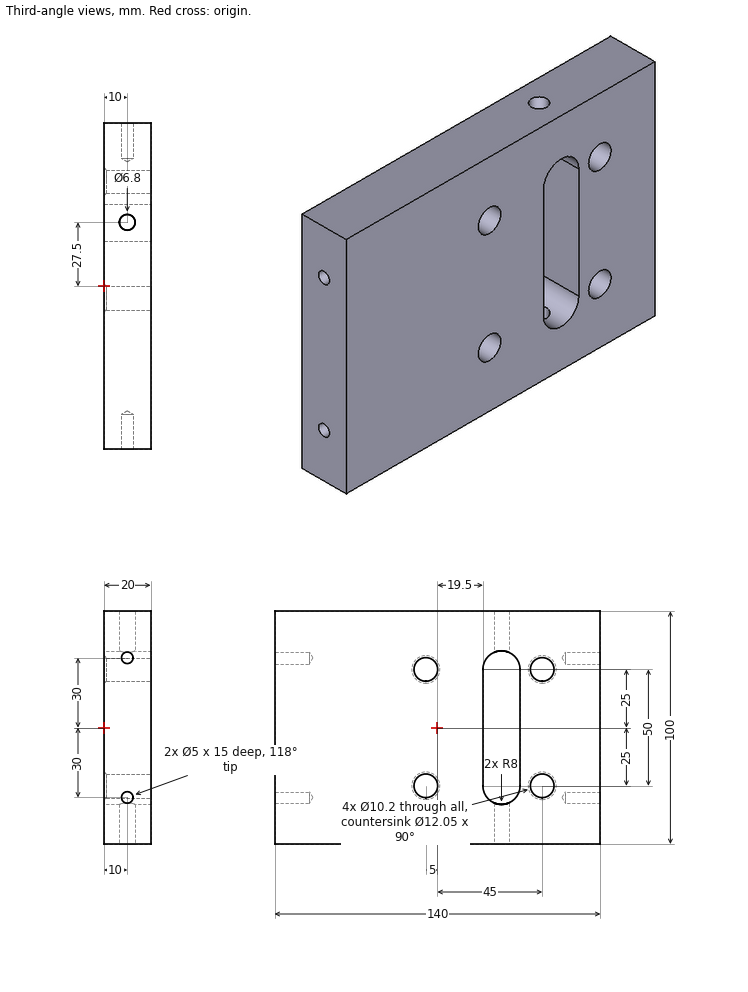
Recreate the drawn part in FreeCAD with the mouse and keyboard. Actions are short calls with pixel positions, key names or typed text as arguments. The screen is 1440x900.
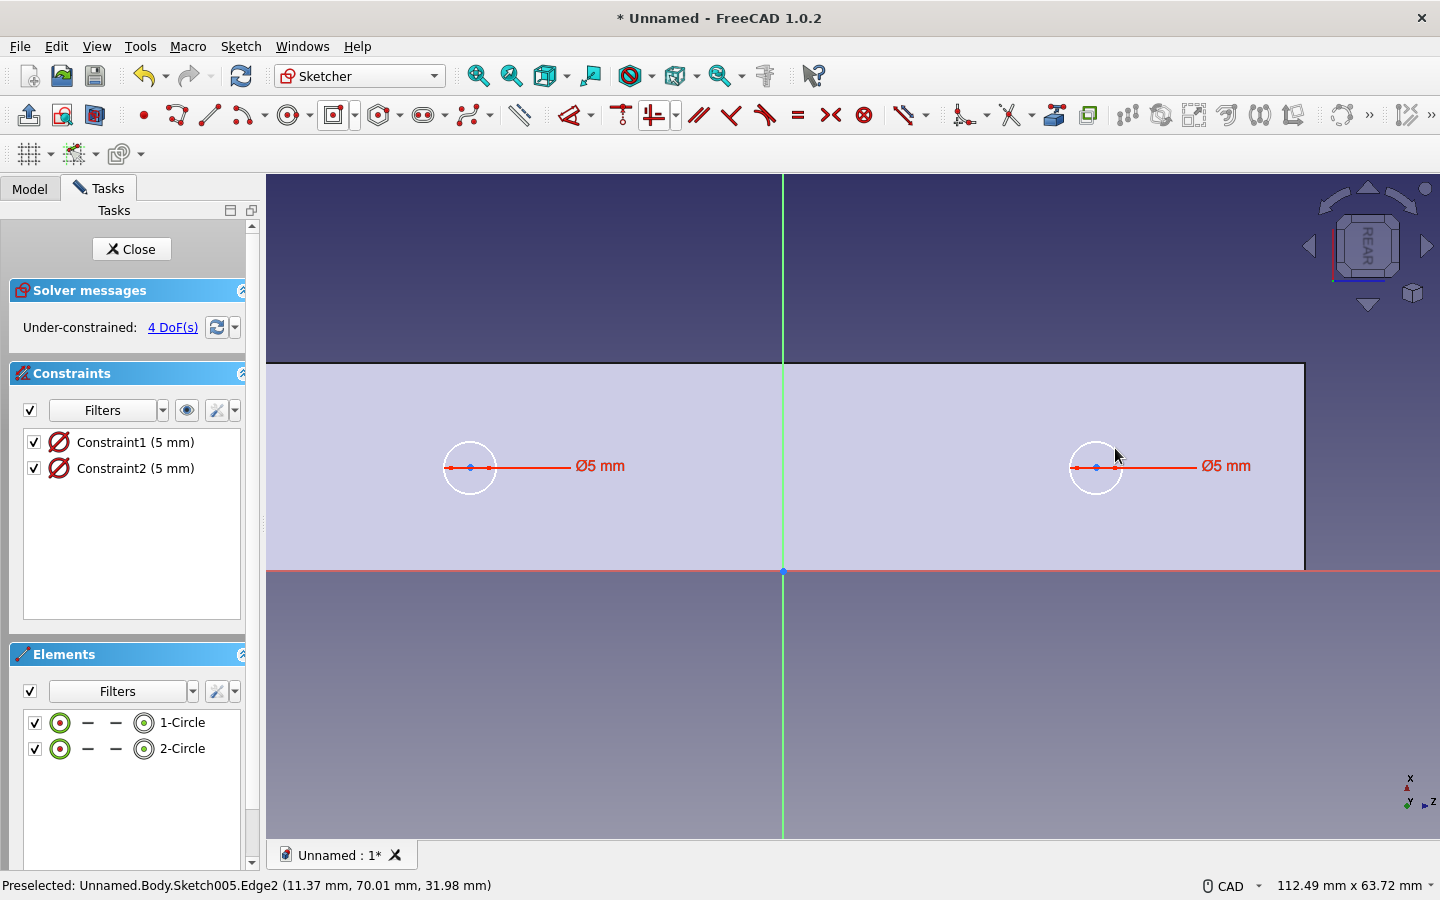
click(470, 468)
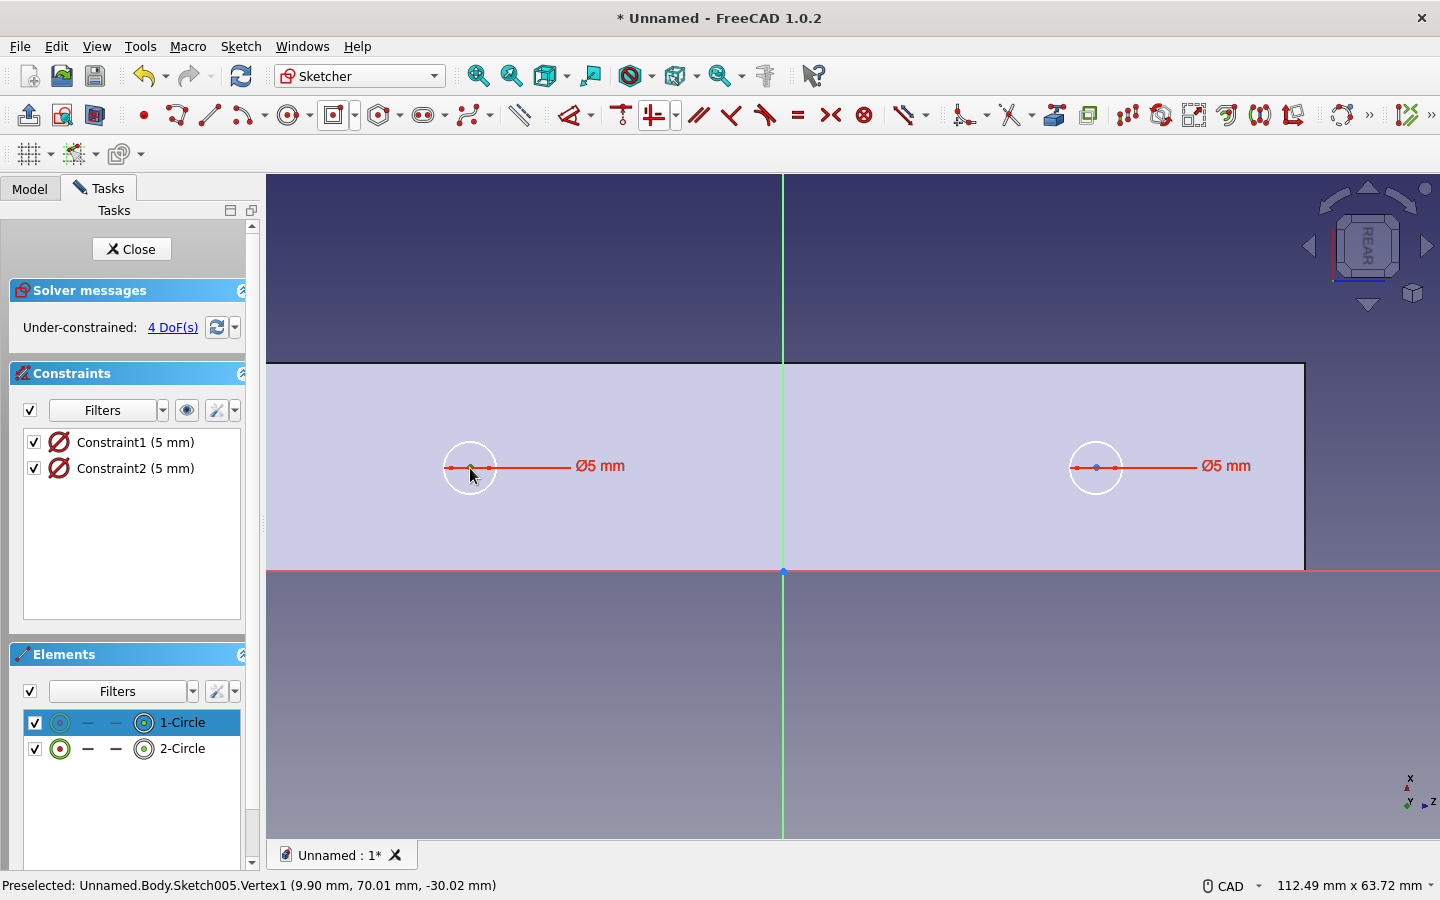
click(1096, 468)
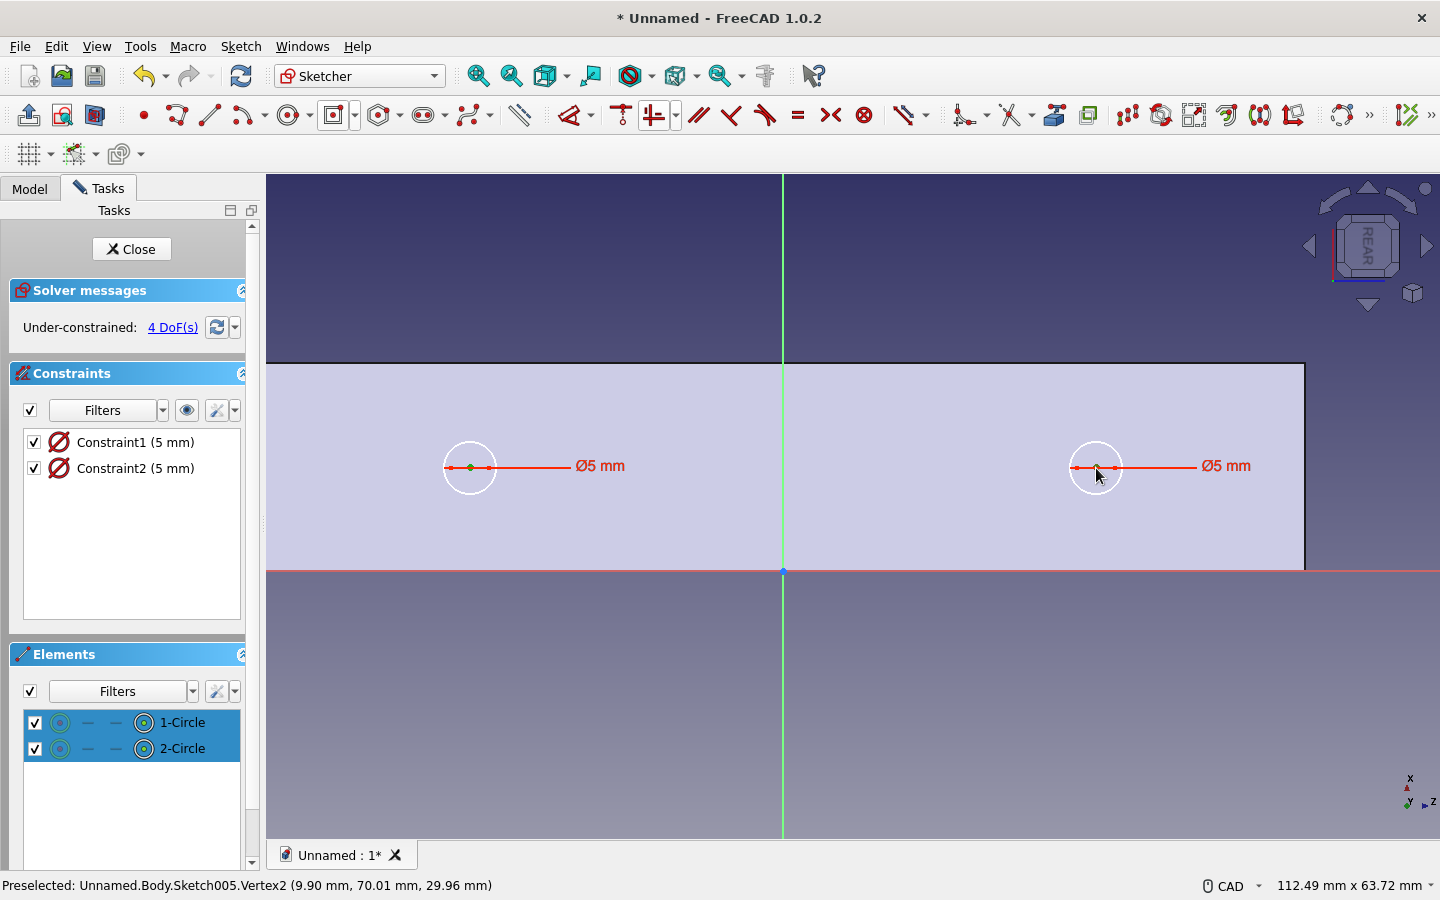
click(676, 116)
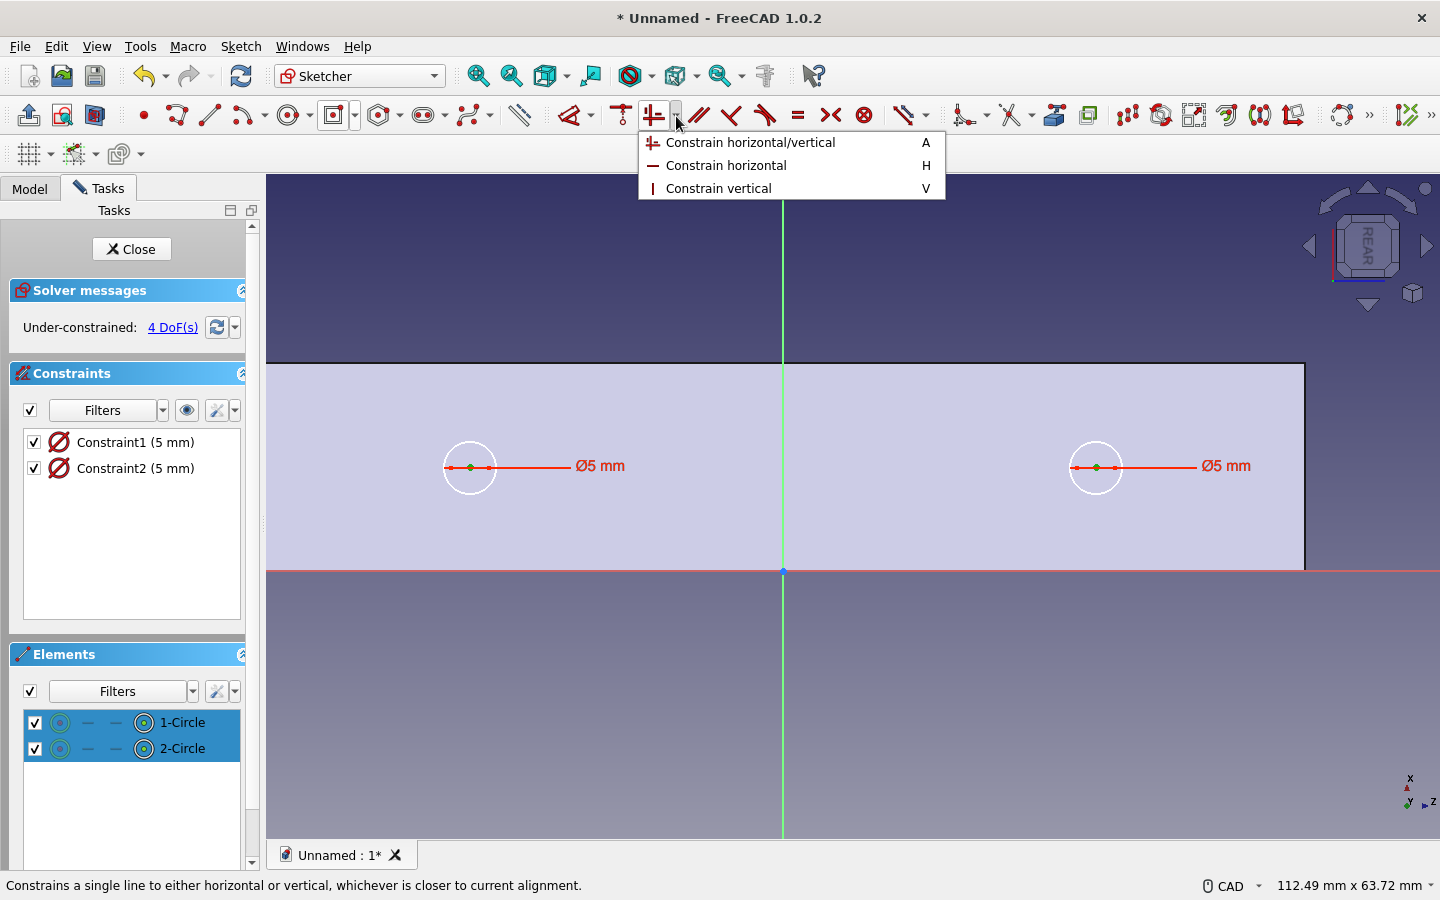
click(792, 166)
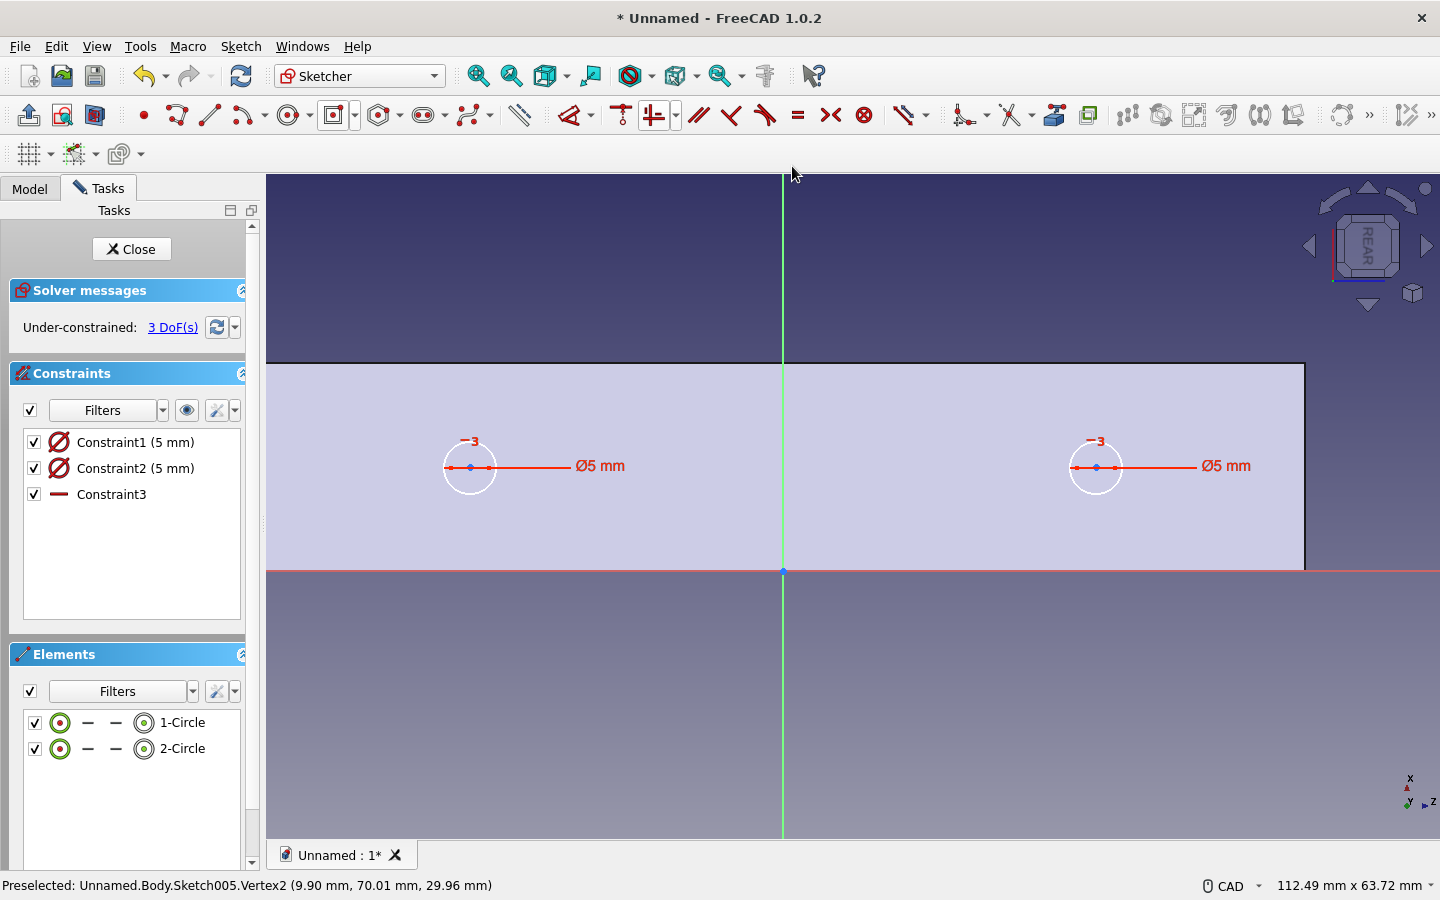
click(568, 116)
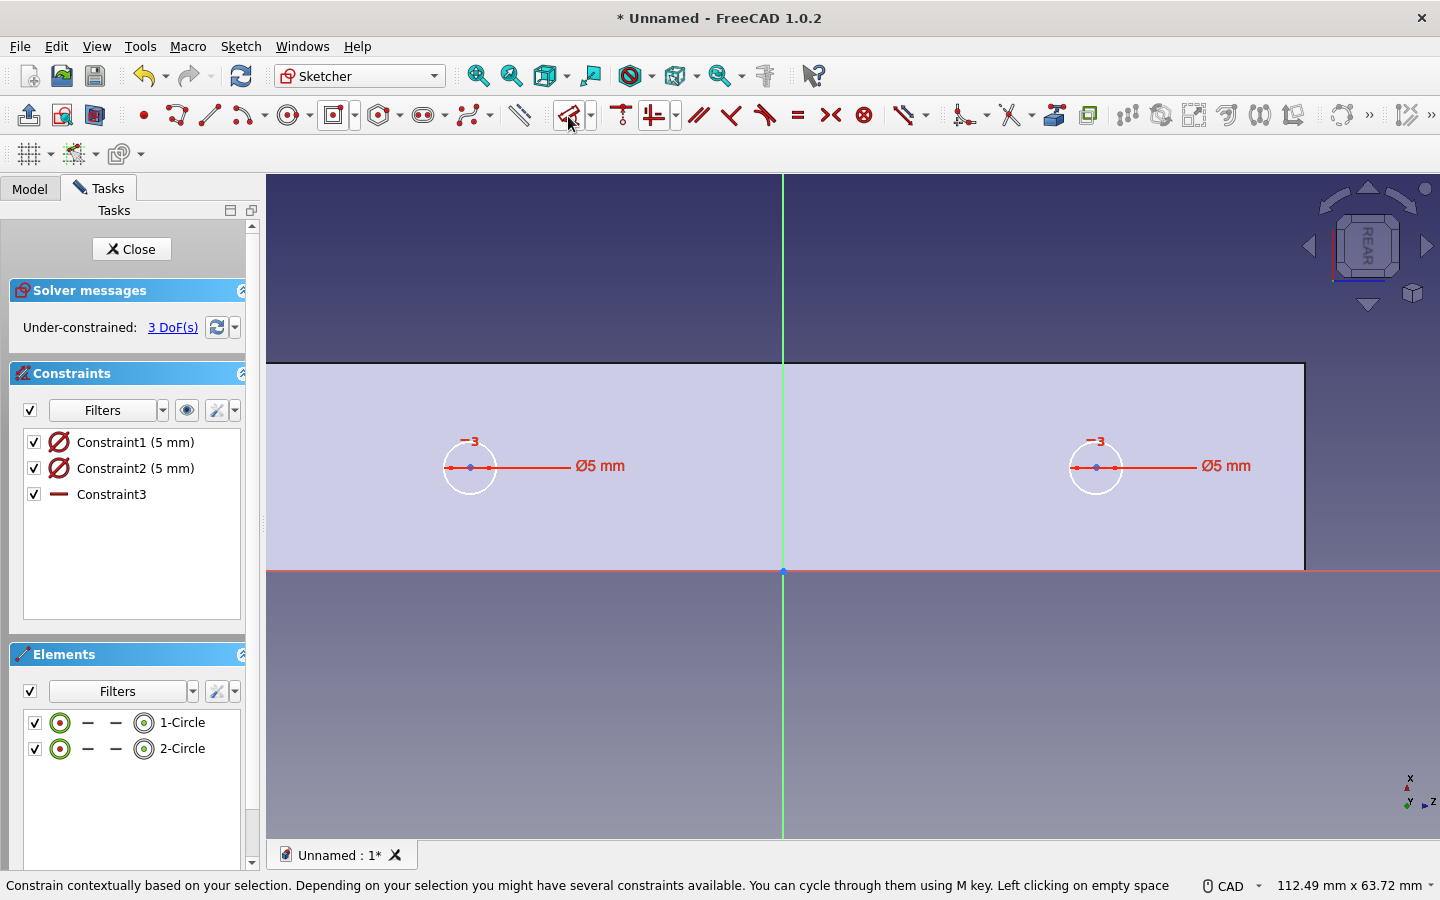
click(470, 468)
click(627, 605)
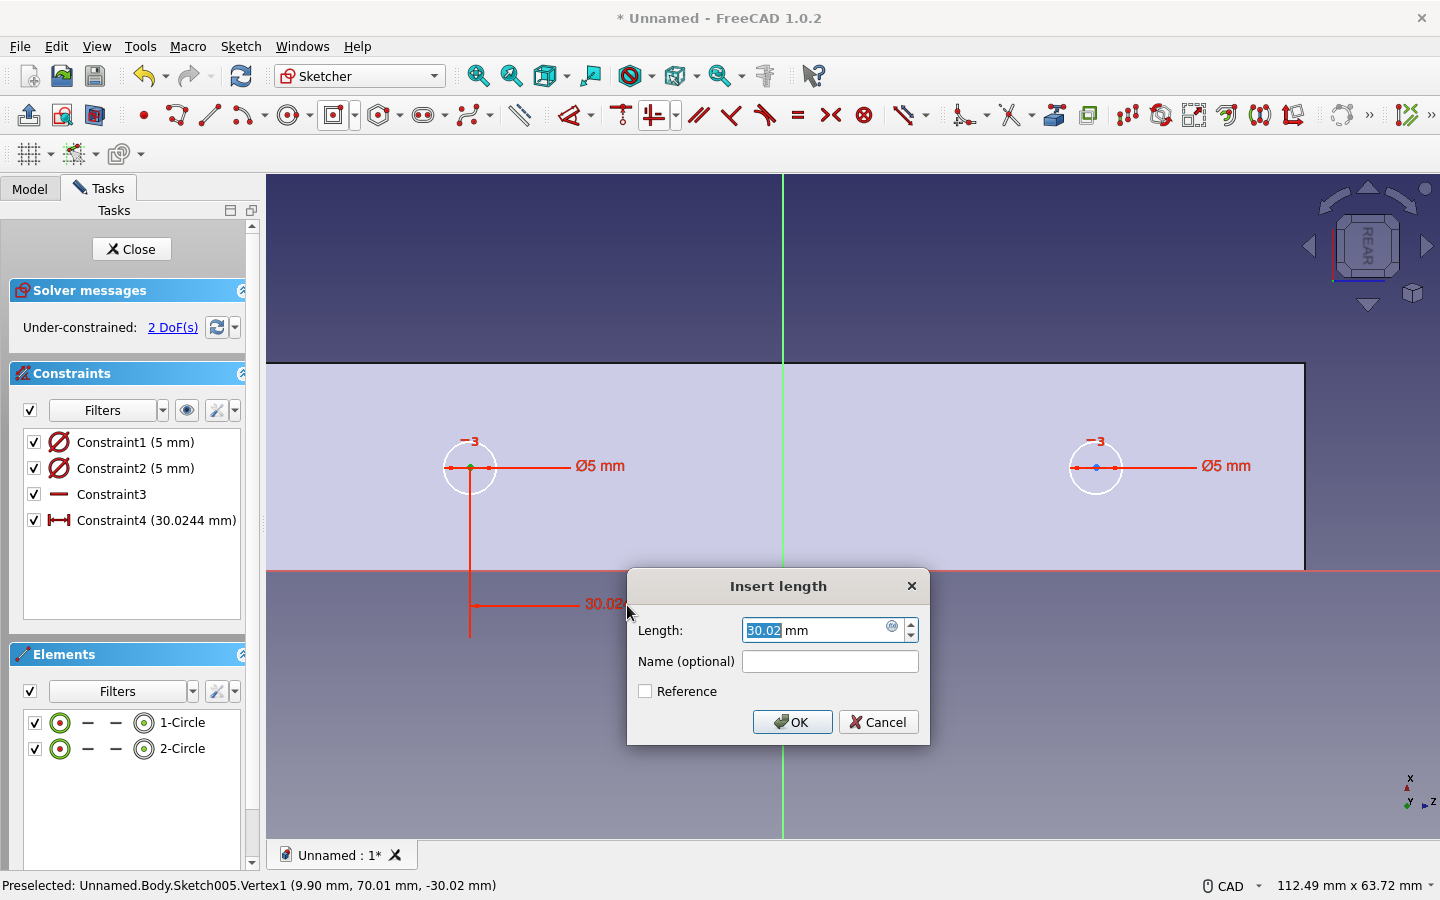
text(30)
key(Return)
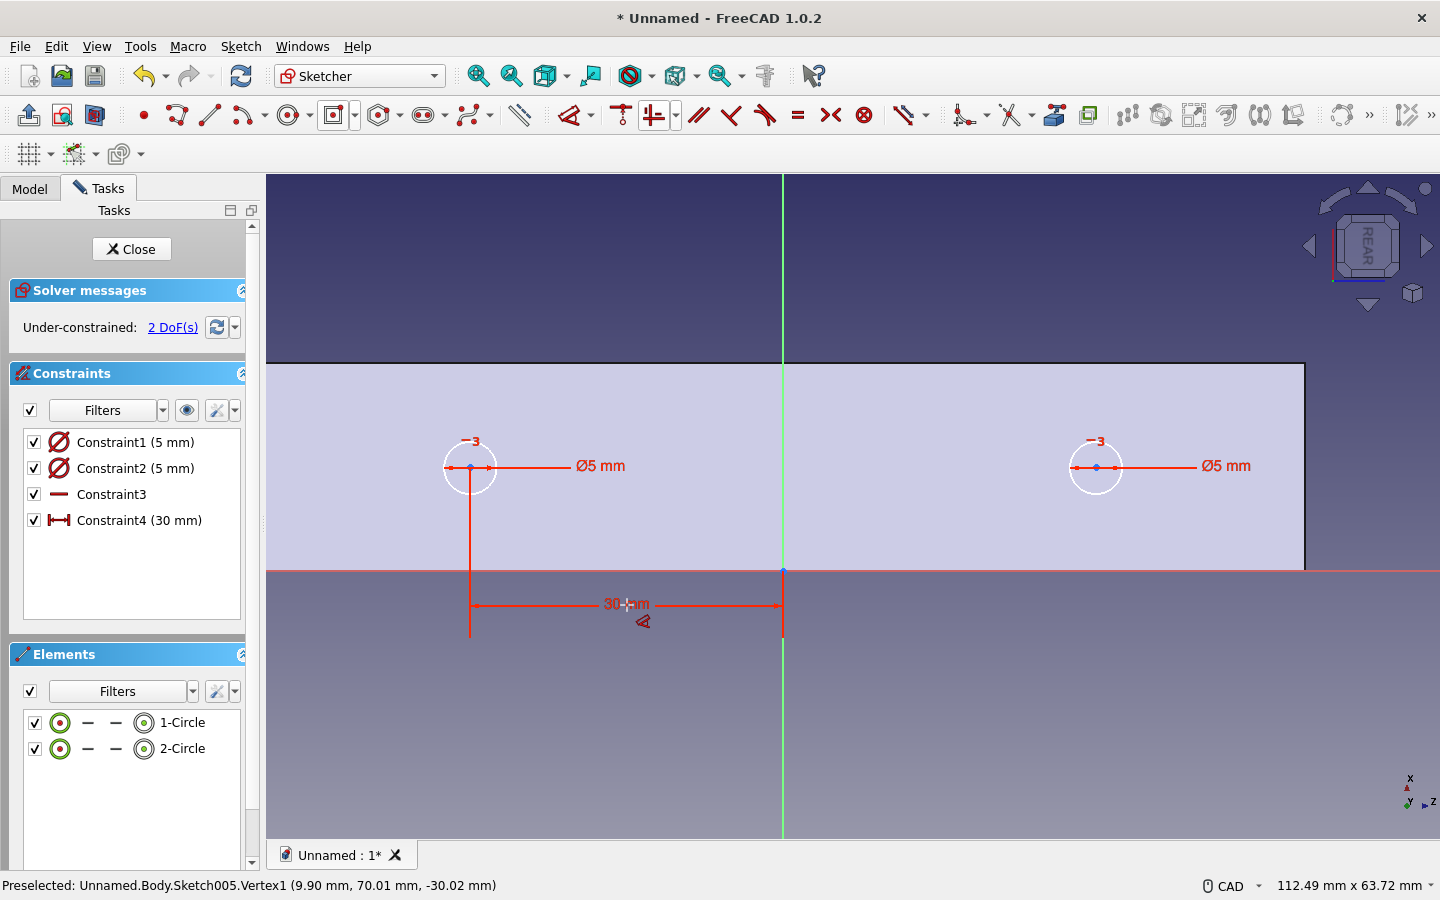
click(470, 468)
click(436, 520)